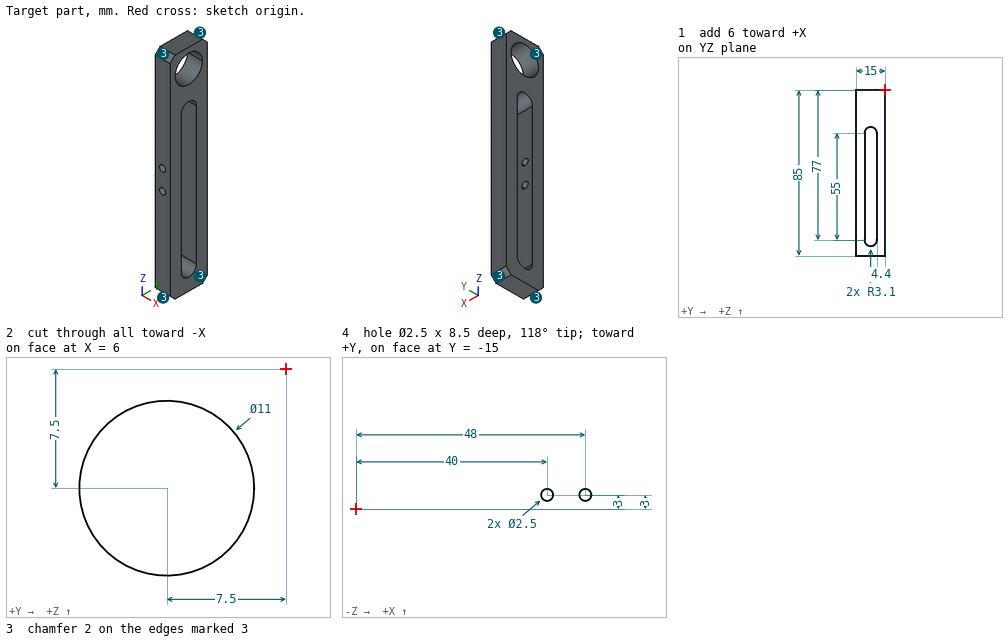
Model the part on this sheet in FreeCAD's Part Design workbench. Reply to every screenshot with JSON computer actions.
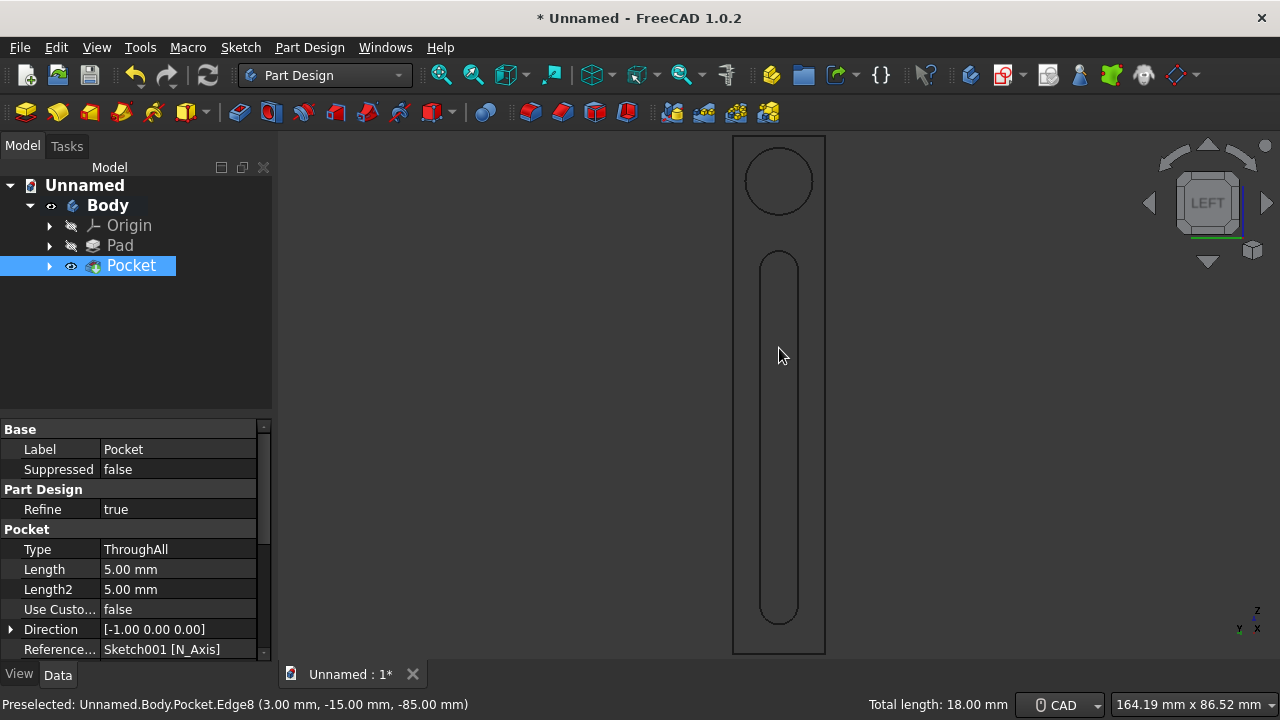
{"action": "key", "text": "0"}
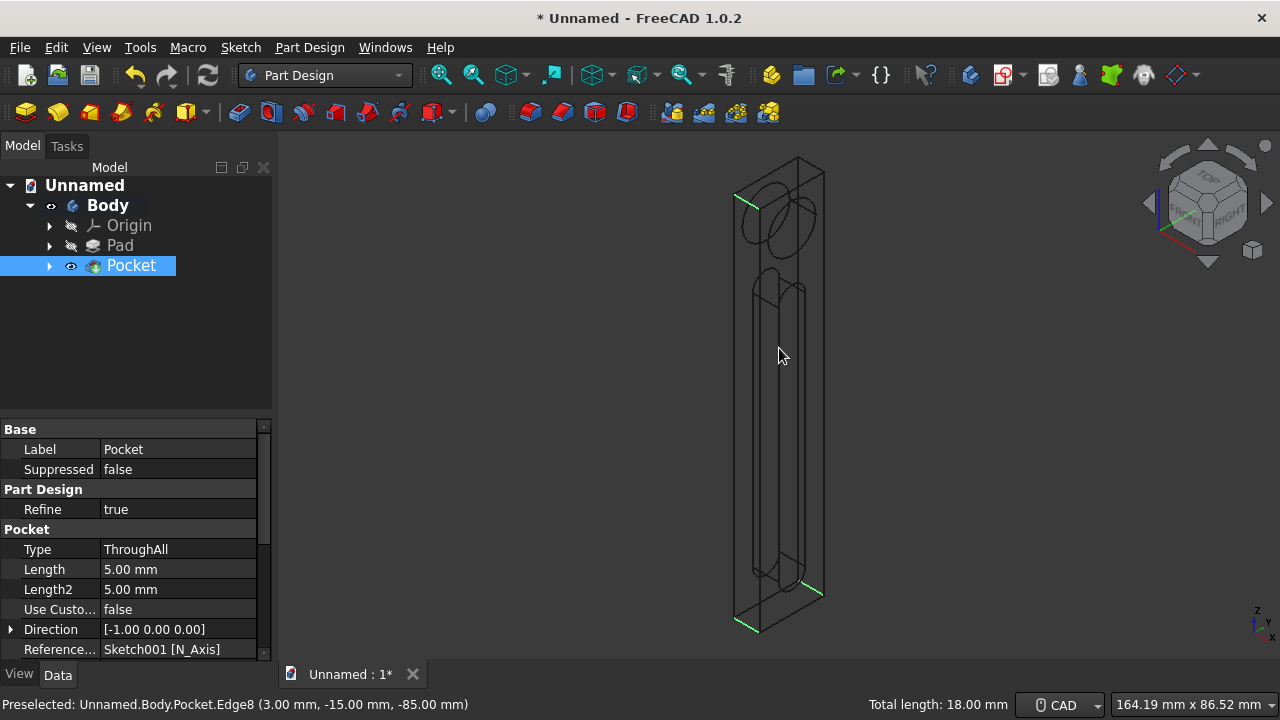
{"action": "left_click", "coordinate": [811, 164], "text": "ctrl"}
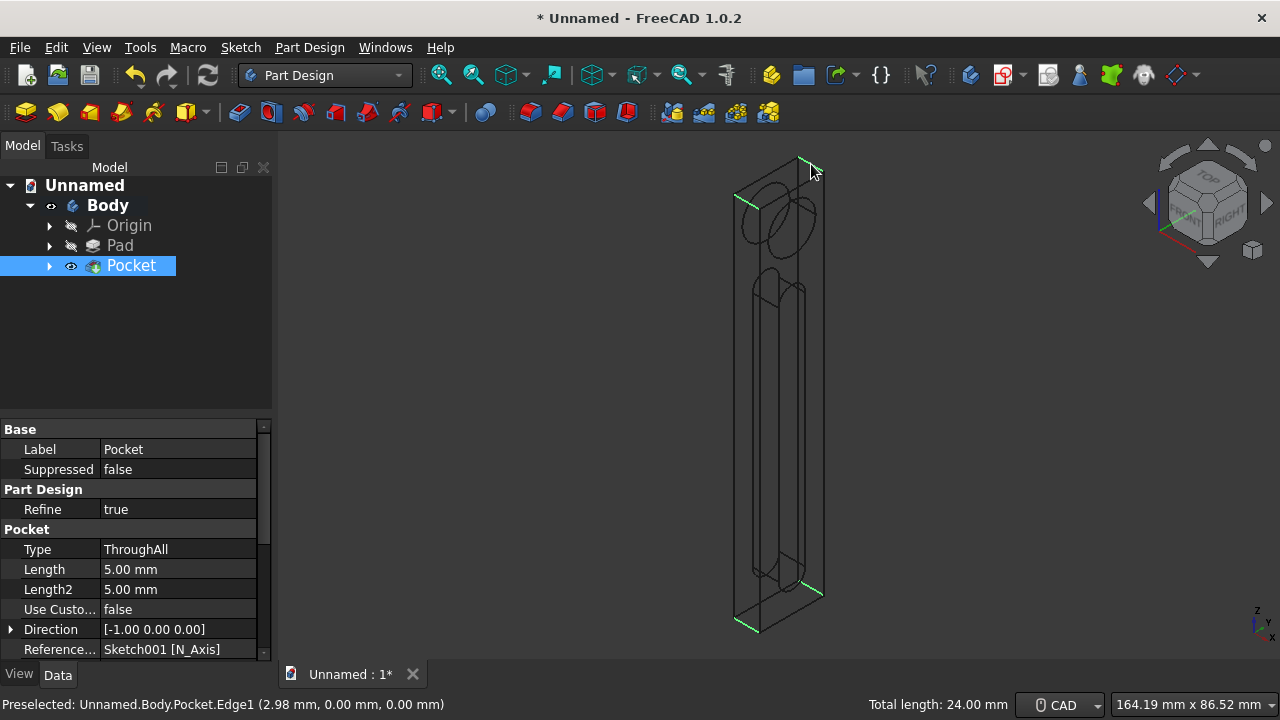
{"action": "key", "text": "v 1"}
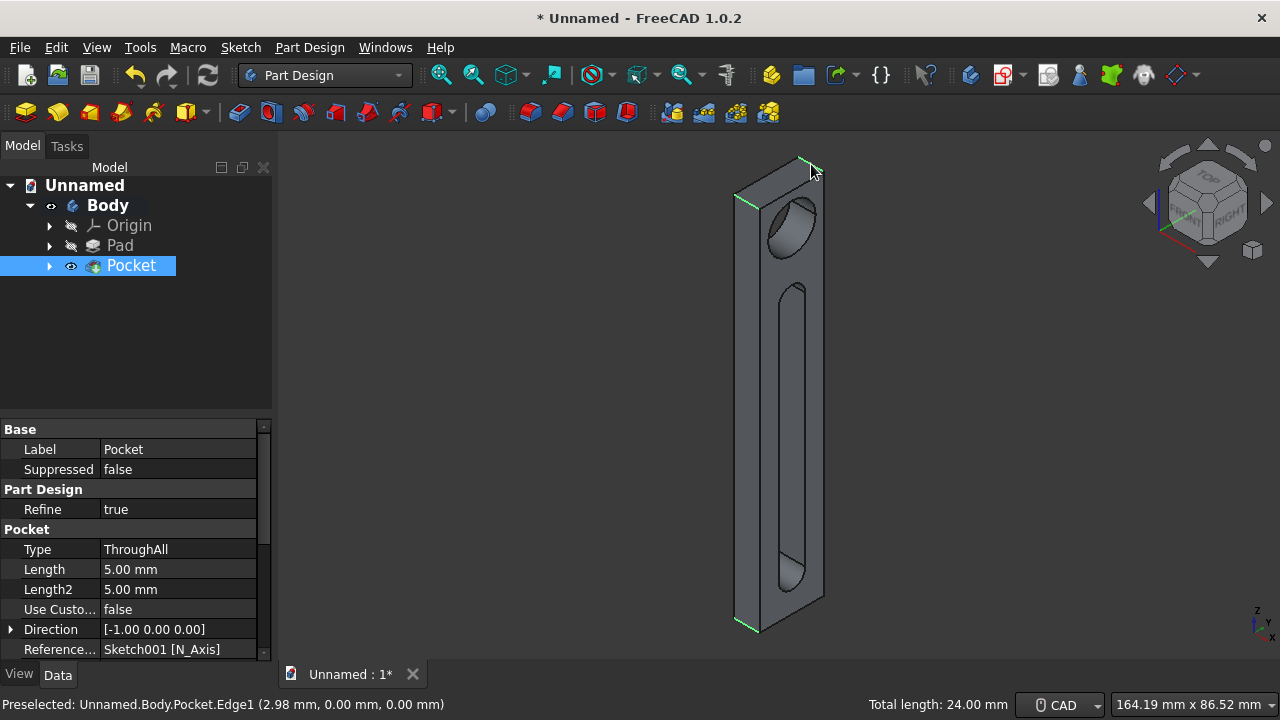
{"action": "left_click", "coordinate": [564, 112]}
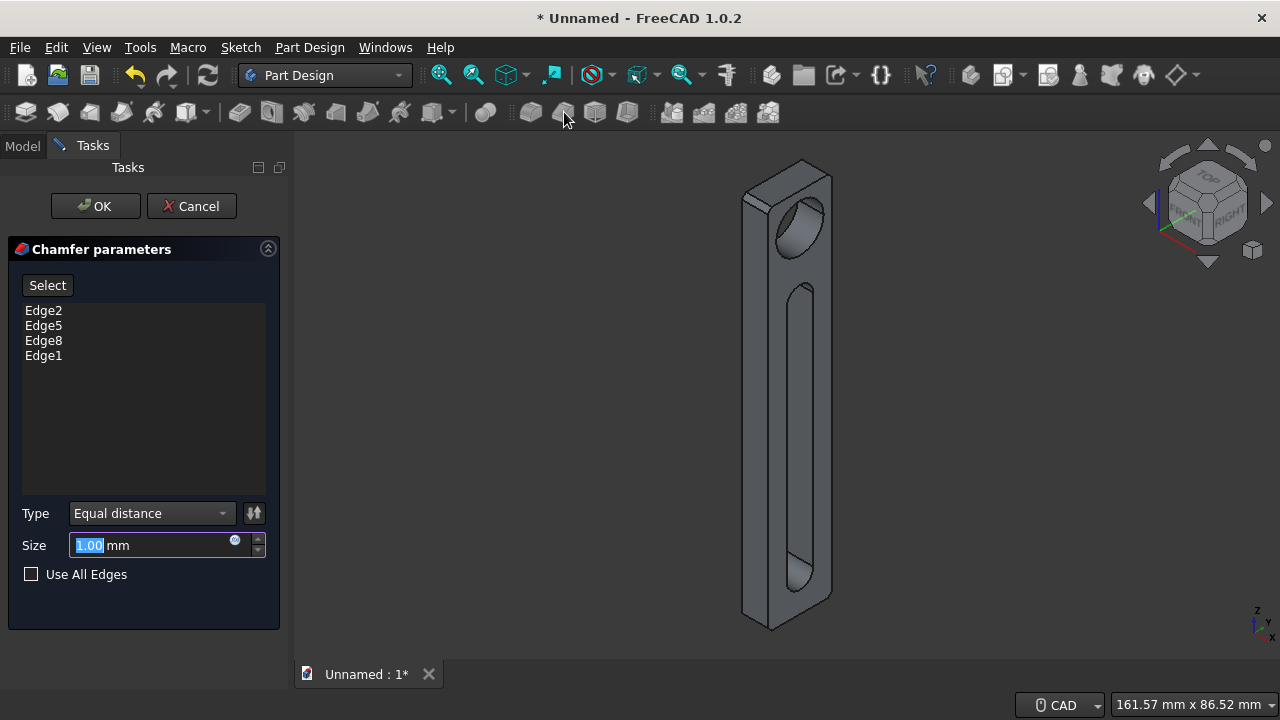
{"action": "type", "text": "2"}
{"action": "key", "text": "Tab"}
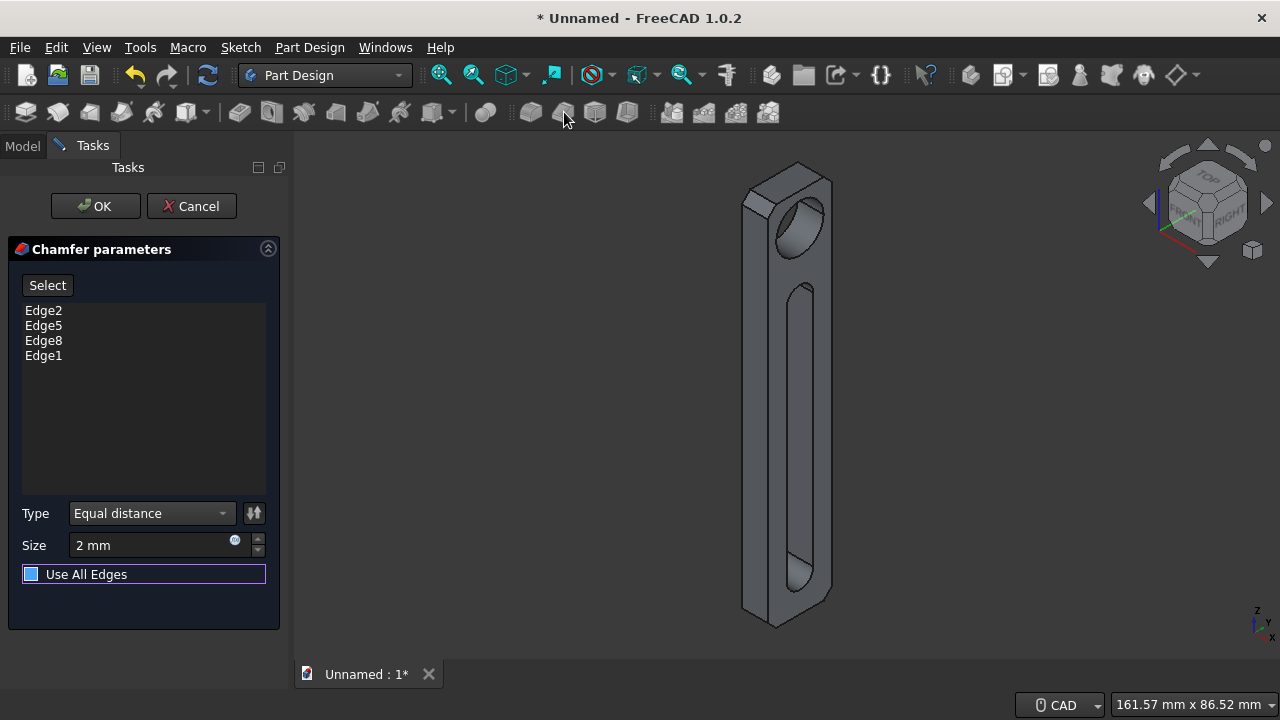
{"action": "left_click", "coordinate": [96, 206]}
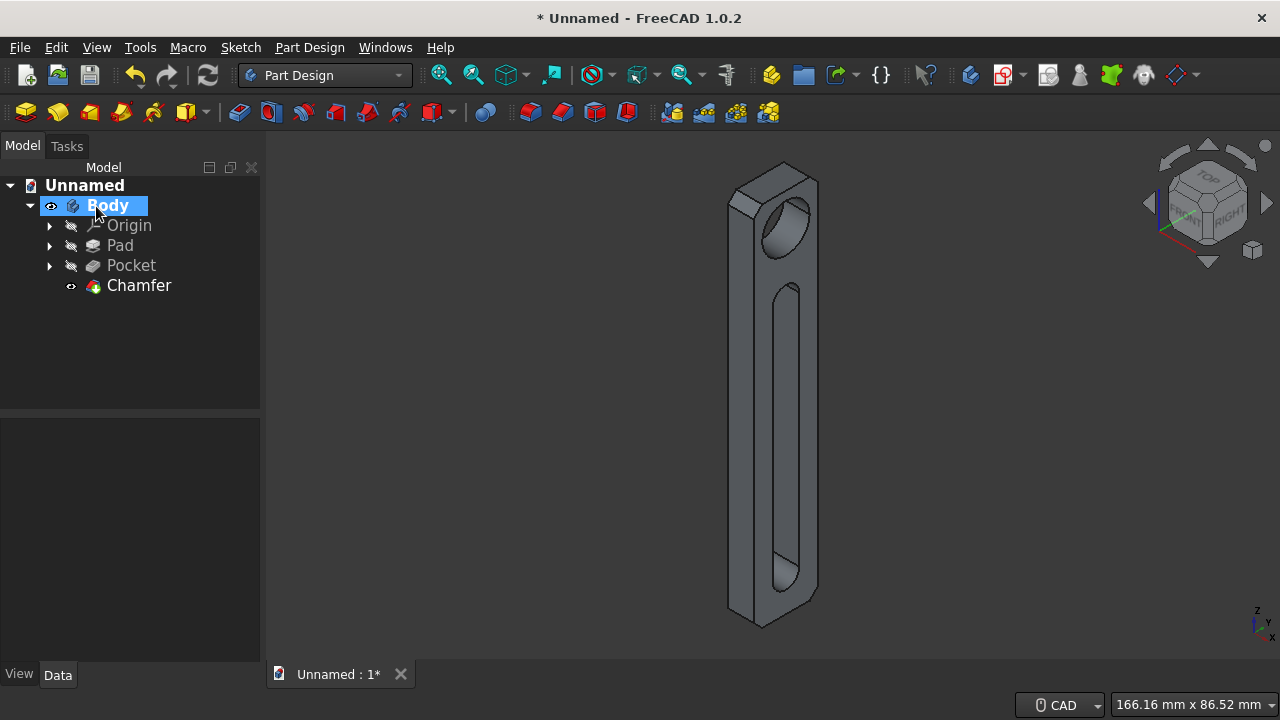
{"action": "left_click", "coordinate": [741, 470]}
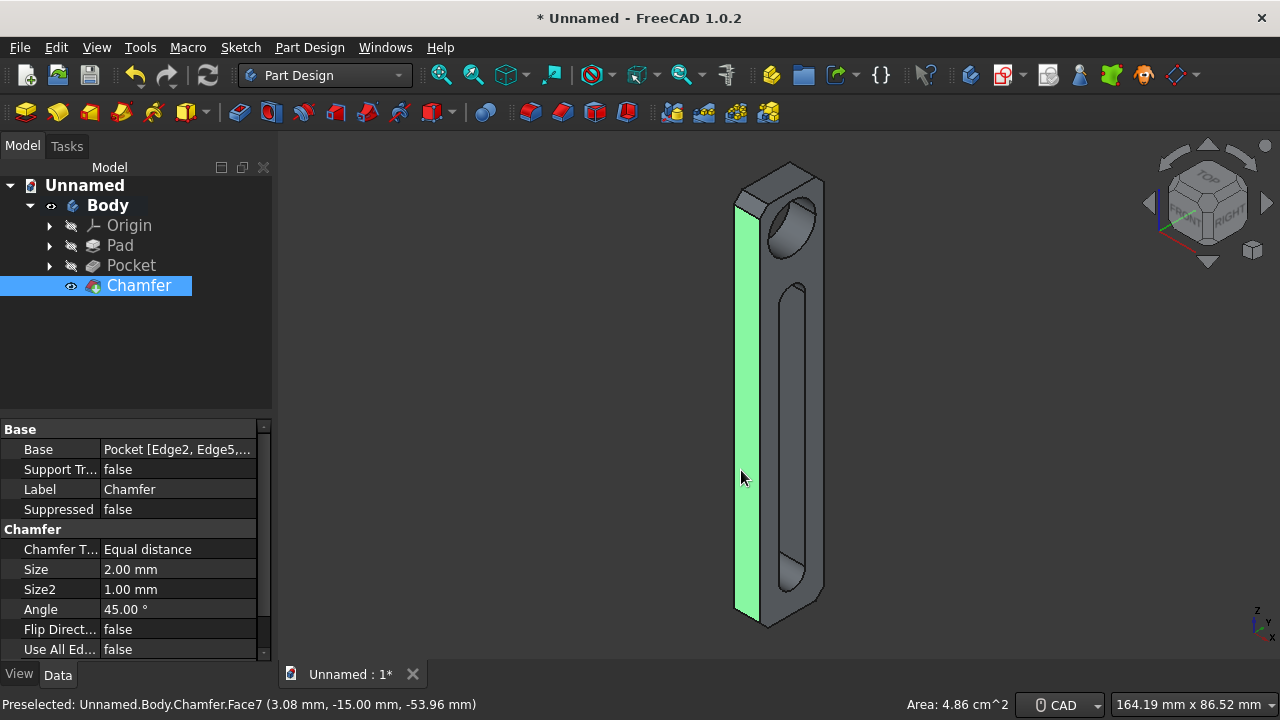
{"action": "left_click", "coordinate": [1004, 76]}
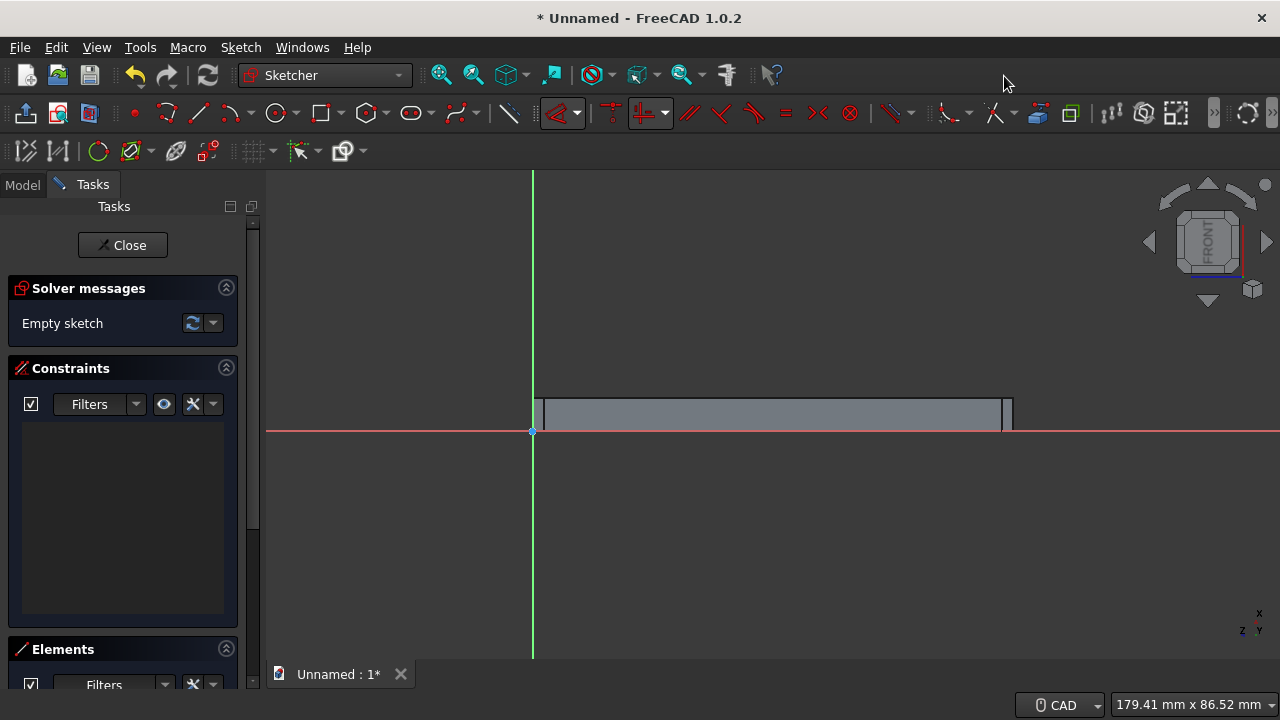
{"action": "scroll", "coordinate": [791, 414], "scroll_direction": "up", "scroll_amount": 11}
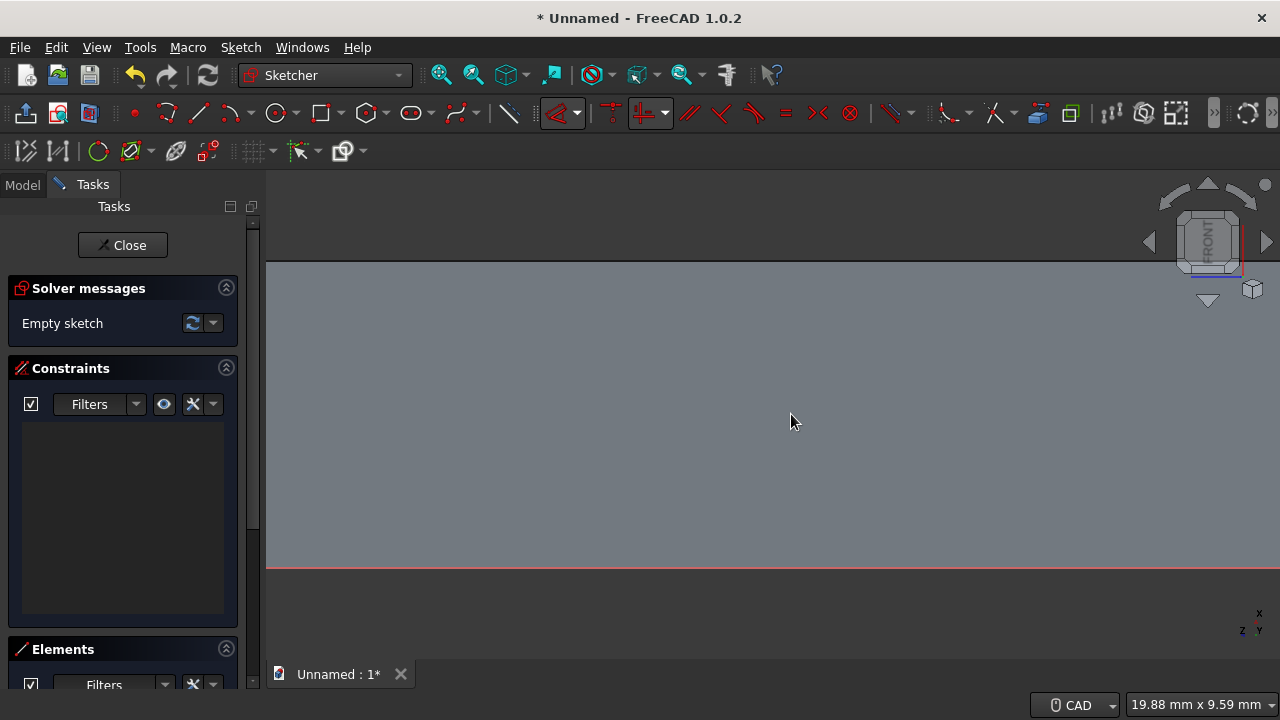
{"action": "left_click", "coordinate": [276, 114]}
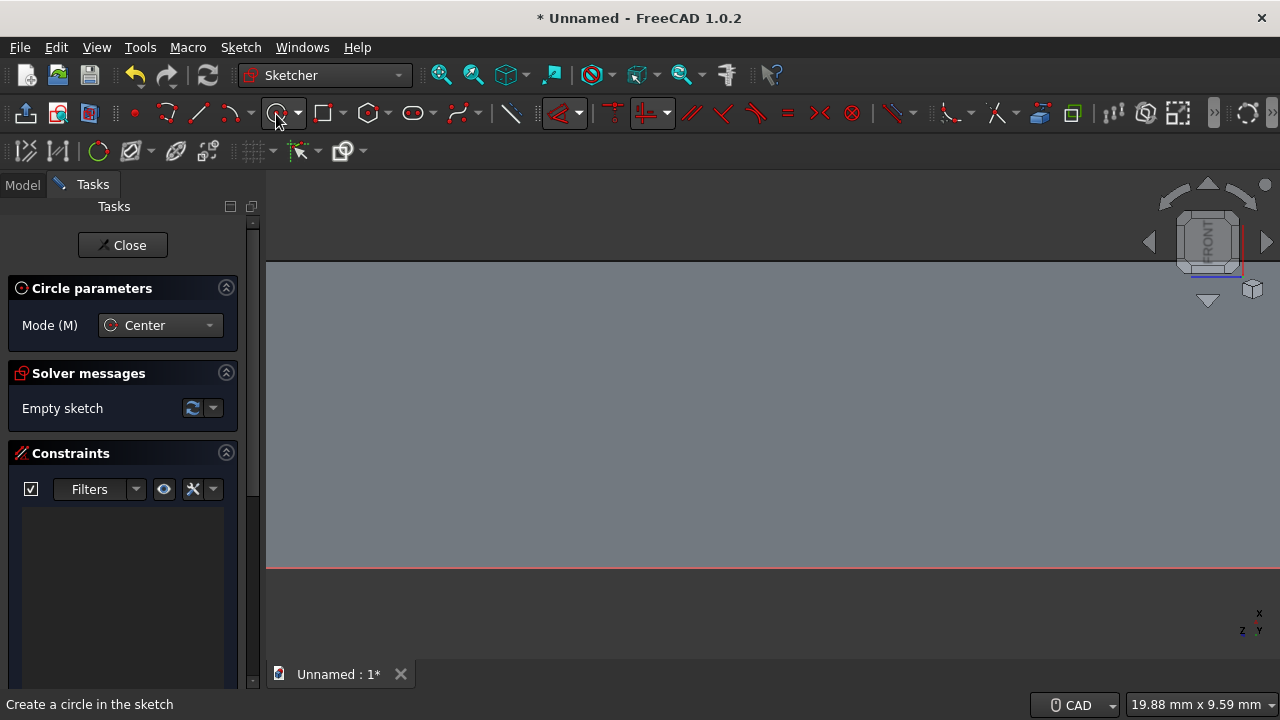
{"action": "left_click", "coordinate": [497, 415]}
{"action": "left_click", "coordinate": [542, 369]}